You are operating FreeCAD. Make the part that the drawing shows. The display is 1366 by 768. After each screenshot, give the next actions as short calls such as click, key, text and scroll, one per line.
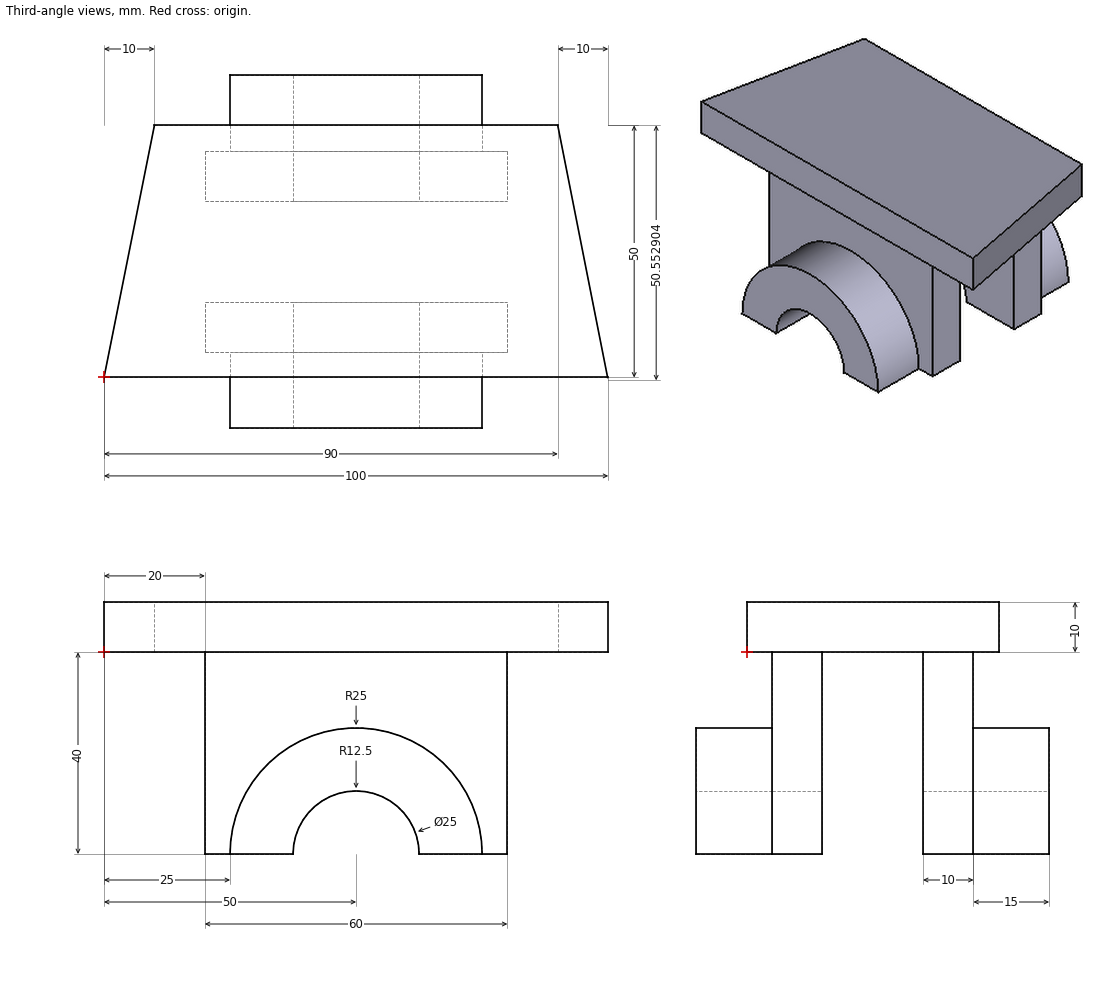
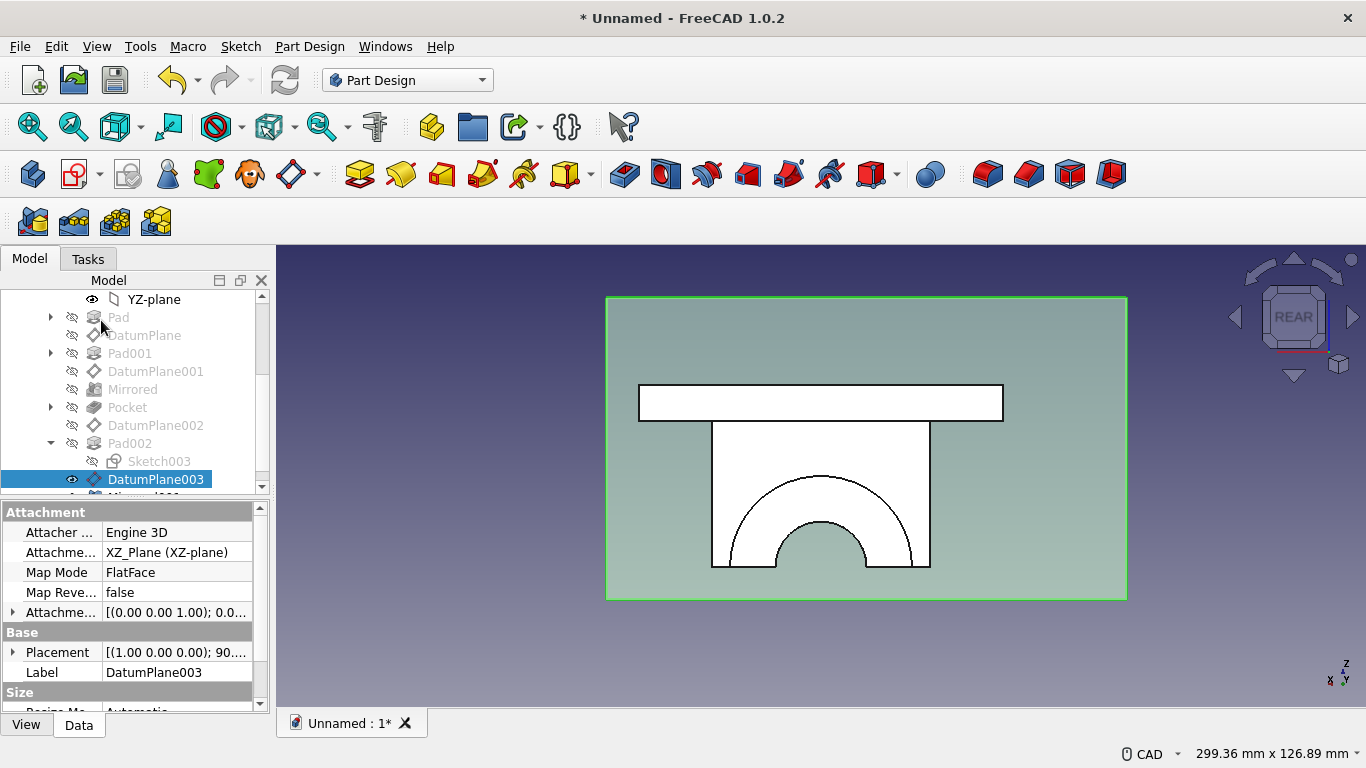
click(117, 479)
key(space)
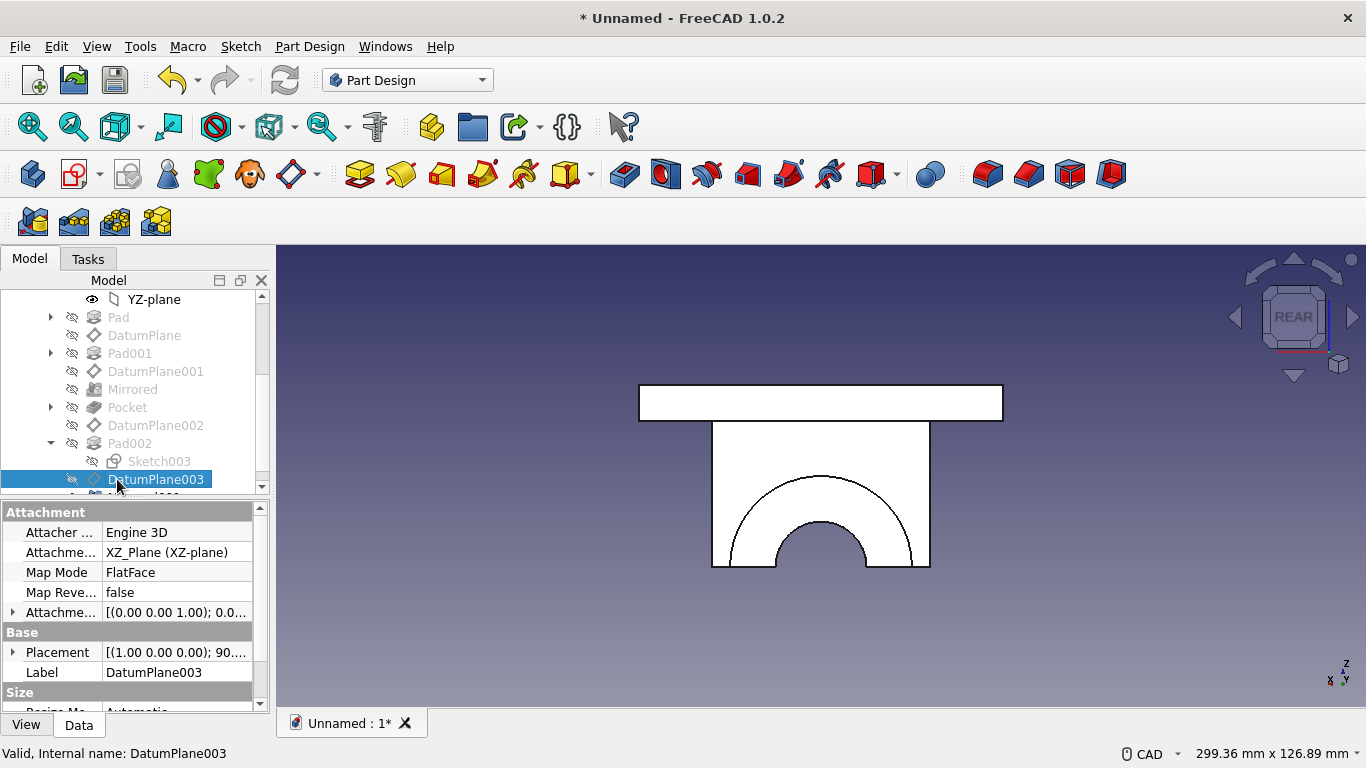
key(v)
key(f)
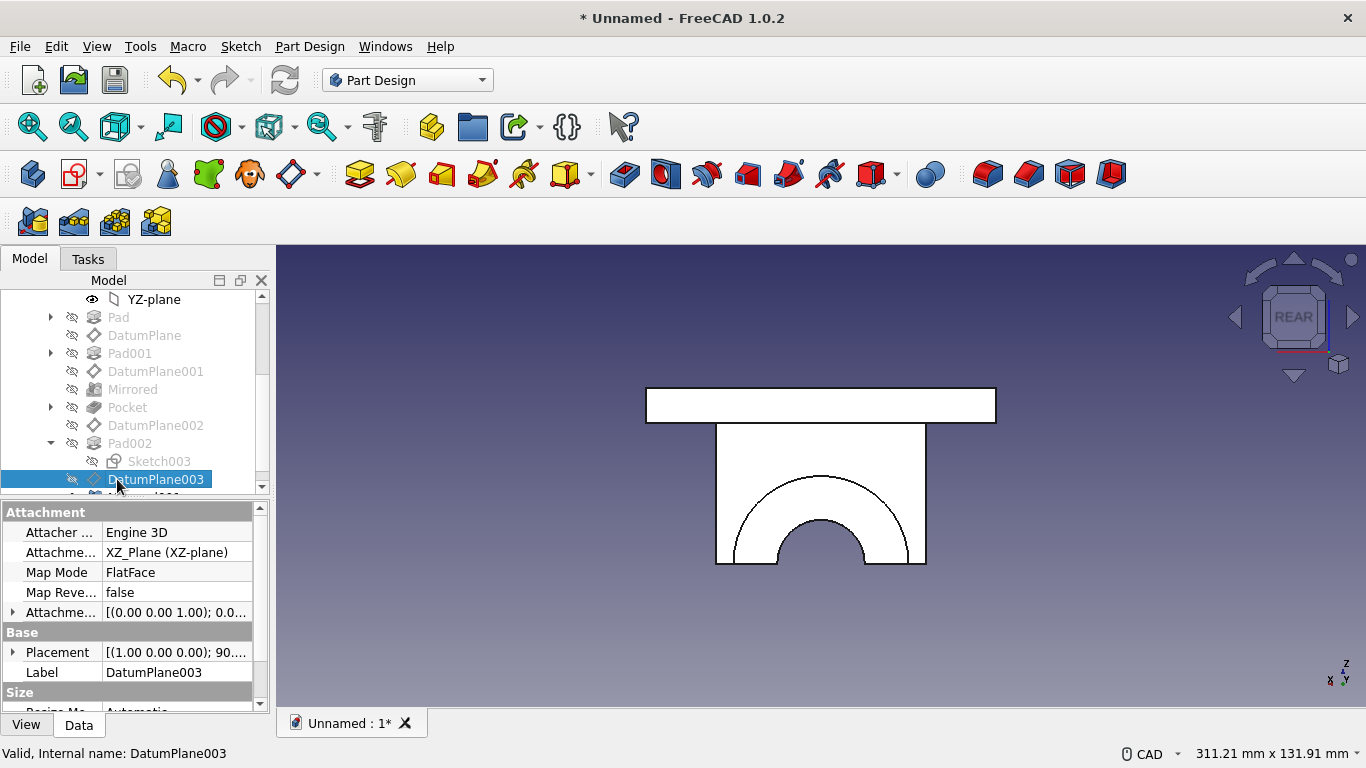
click(316, 667)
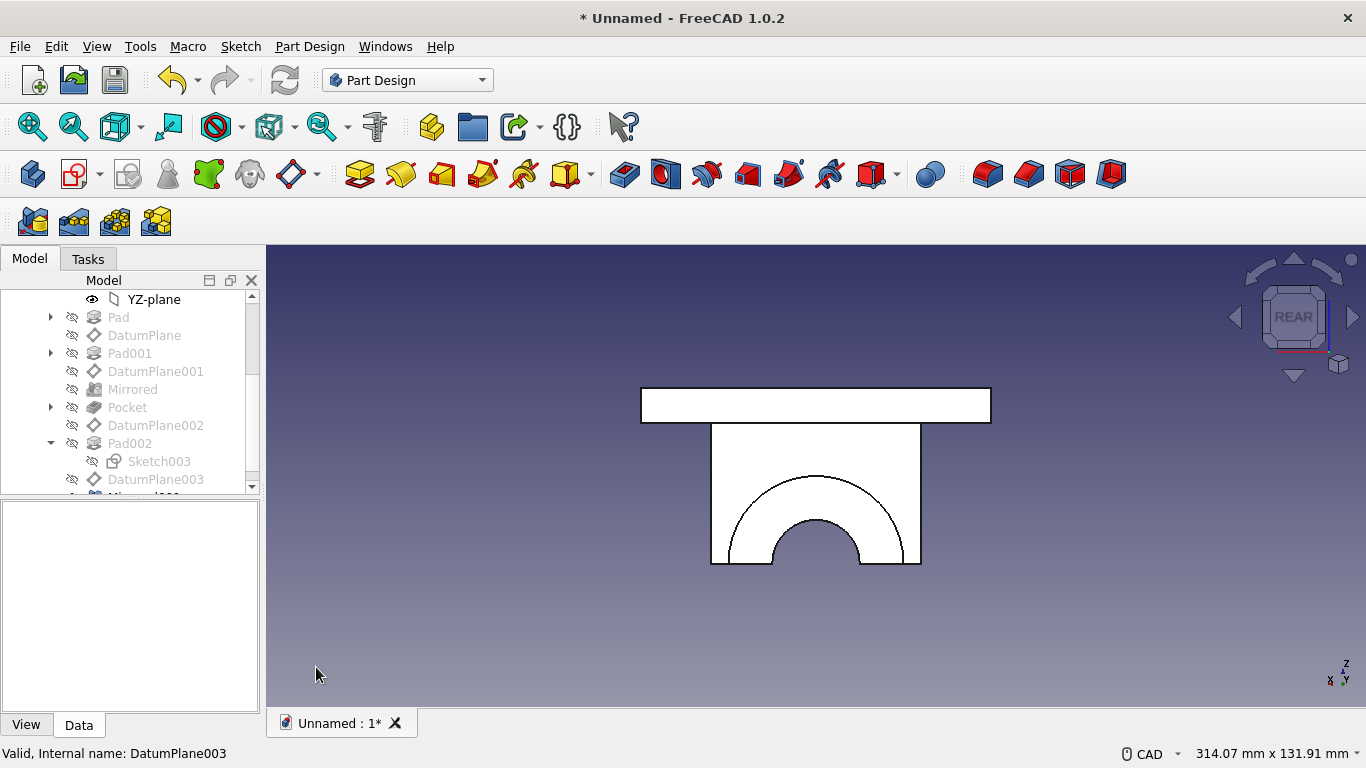
click(74, 174)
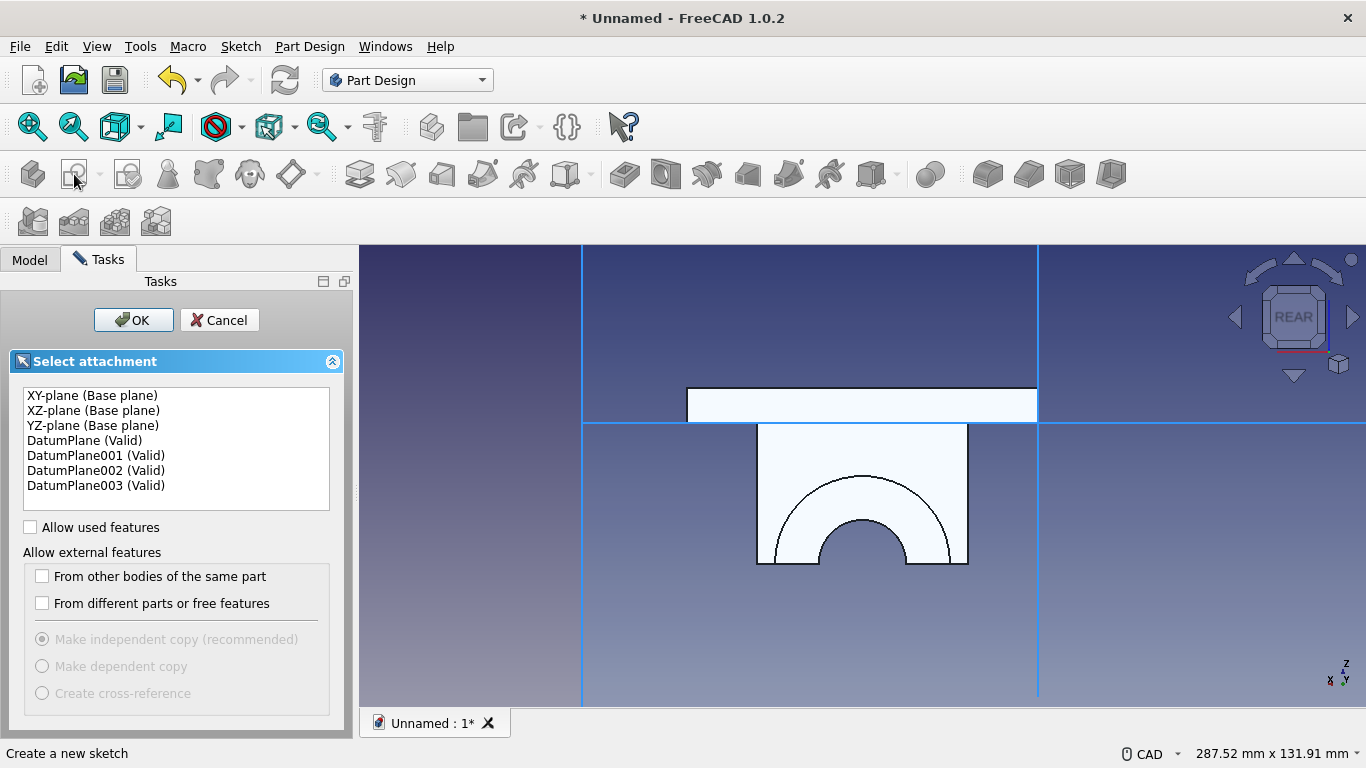
click(84, 396)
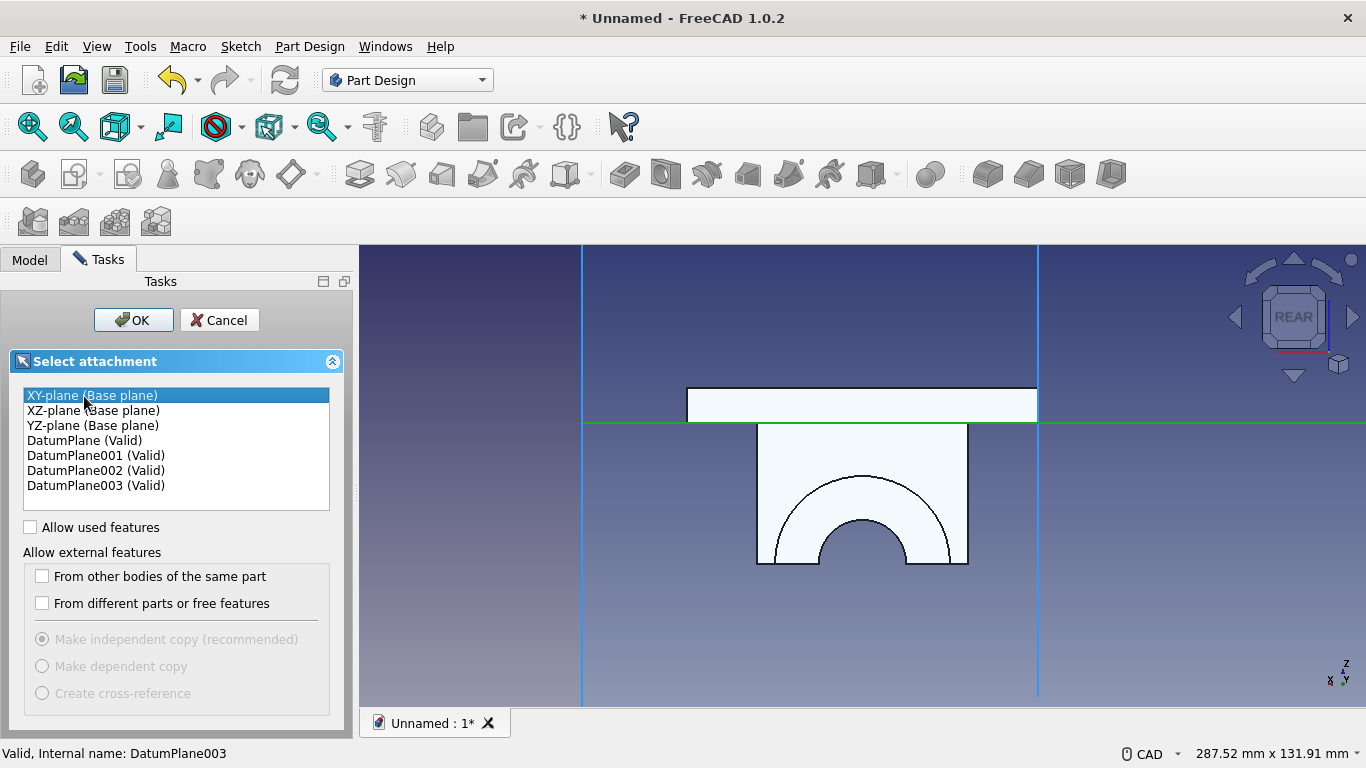
click(134, 320)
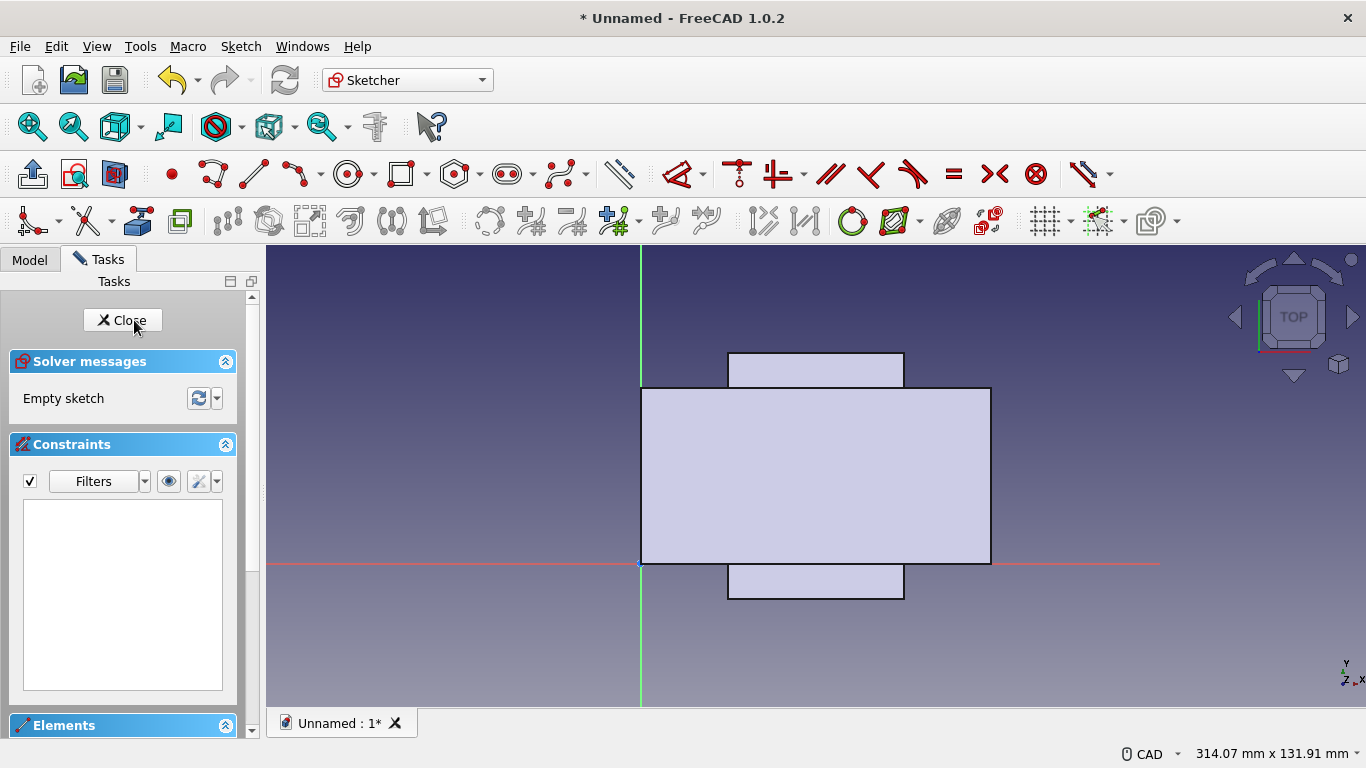
click(115, 174)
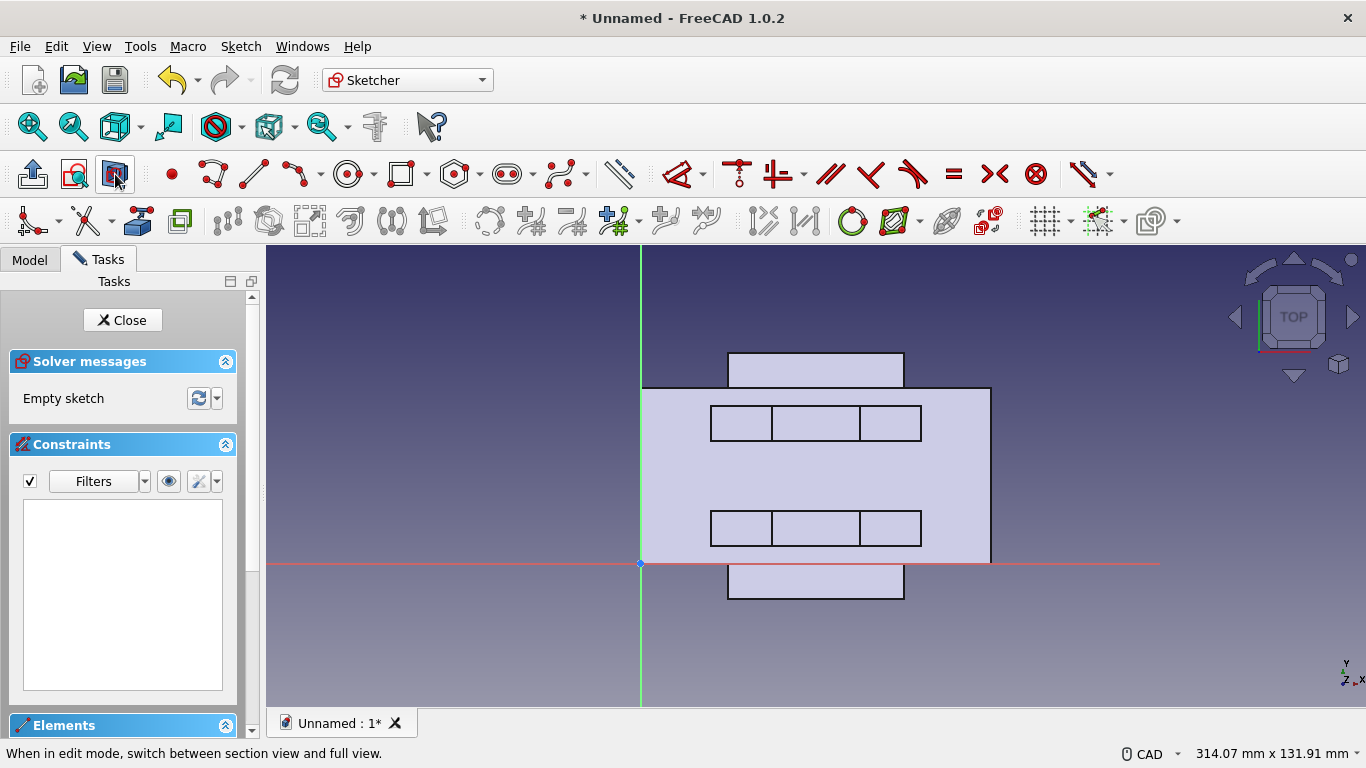
scroll(955, 479, up, 2)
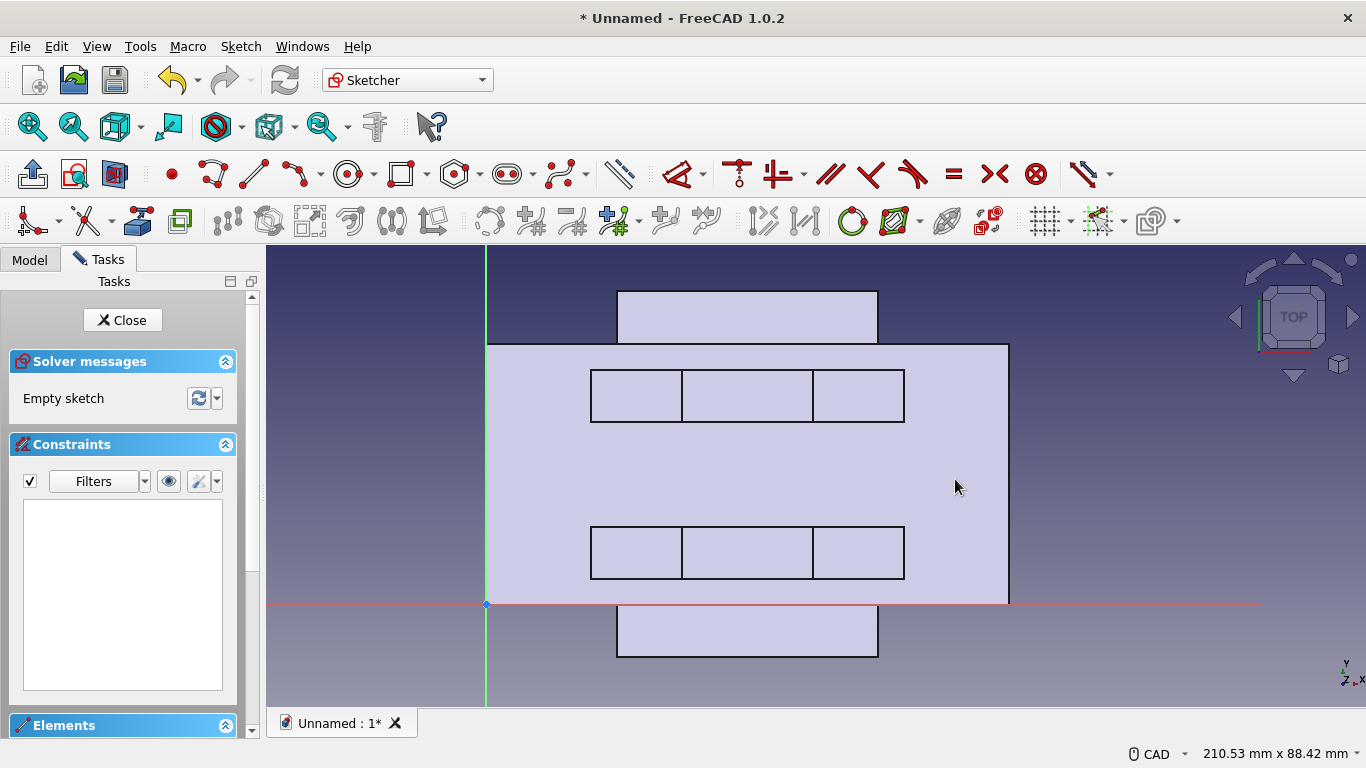
key(g)
key(m)